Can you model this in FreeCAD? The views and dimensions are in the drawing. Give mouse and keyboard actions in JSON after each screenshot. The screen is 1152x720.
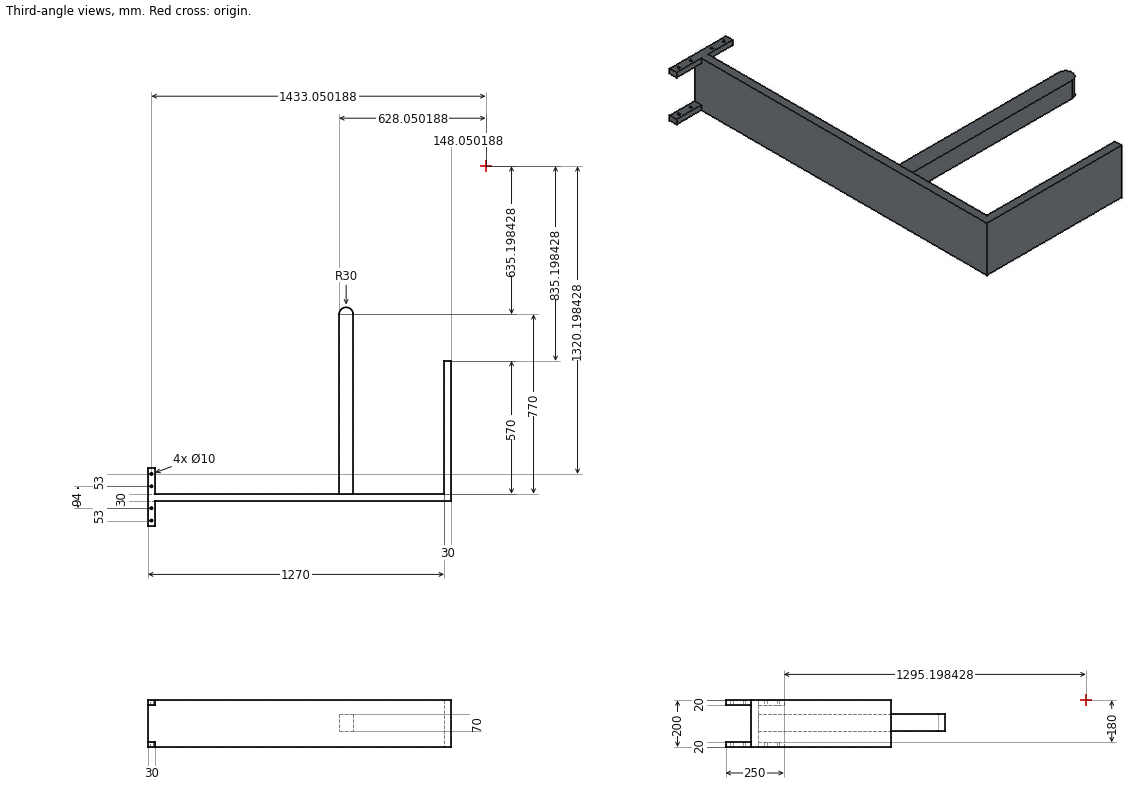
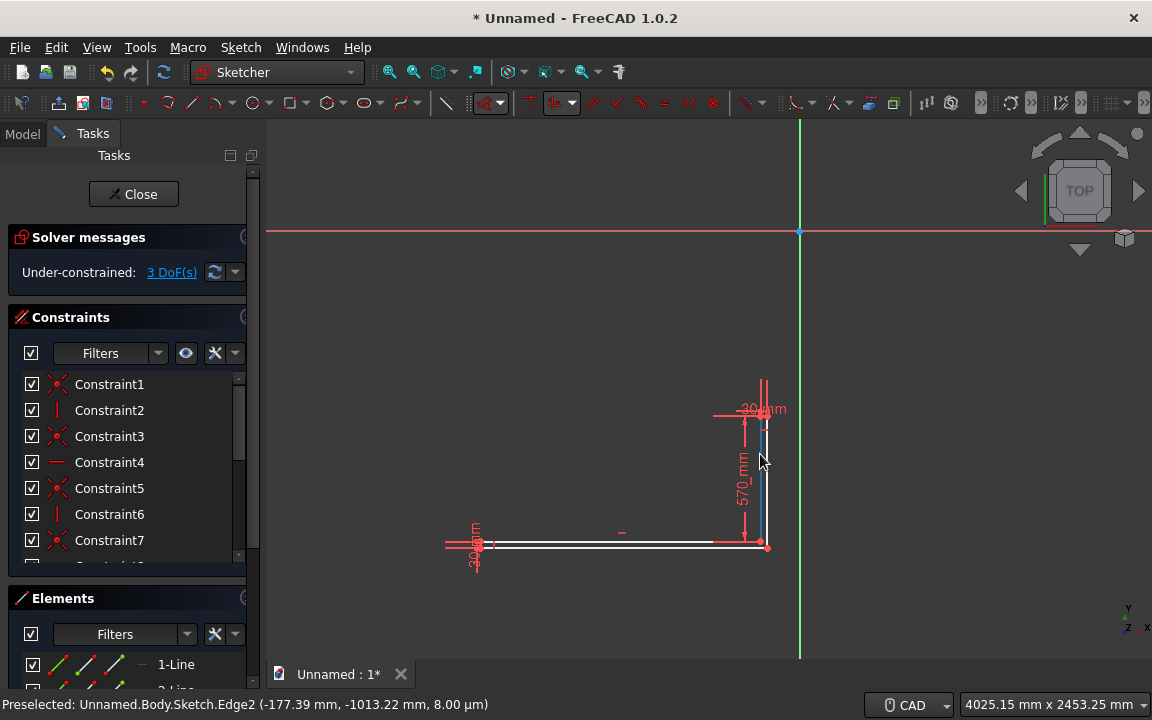
{"action": "scroll", "coordinate": [677, 542], "scroll_direction": "up", "scroll_amount": 4}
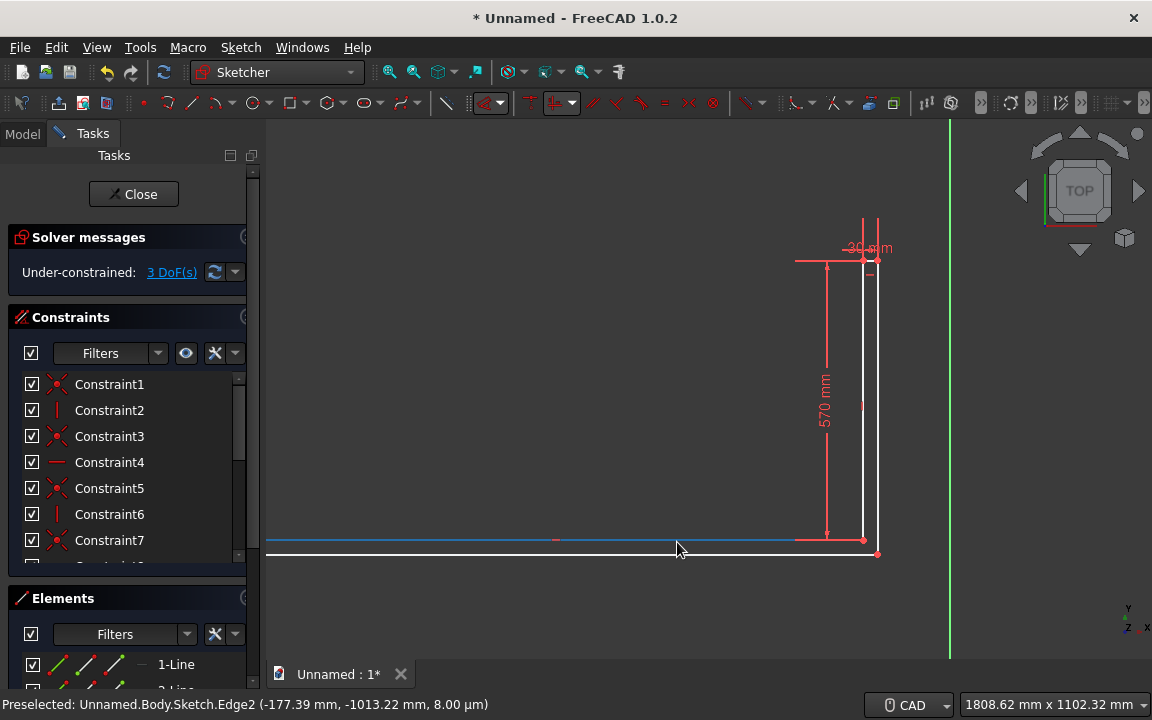
{"action": "left_click", "coordinate": [676, 540]}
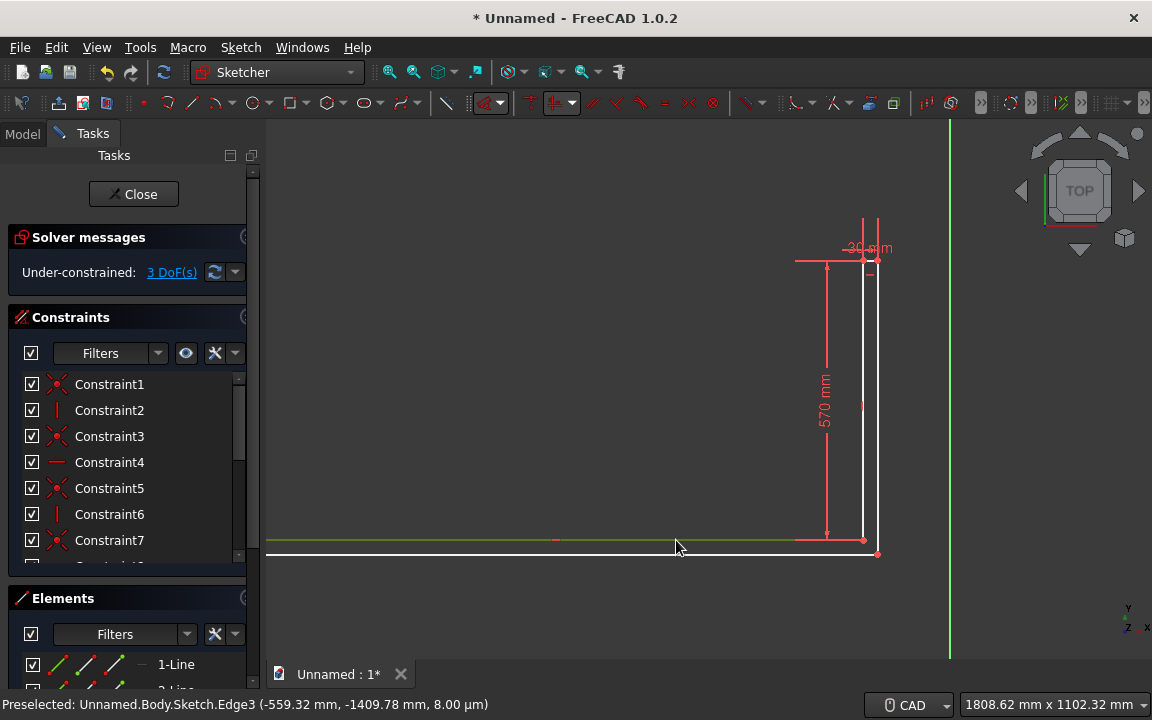
{"action": "left_click", "coordinate": [502, 104]}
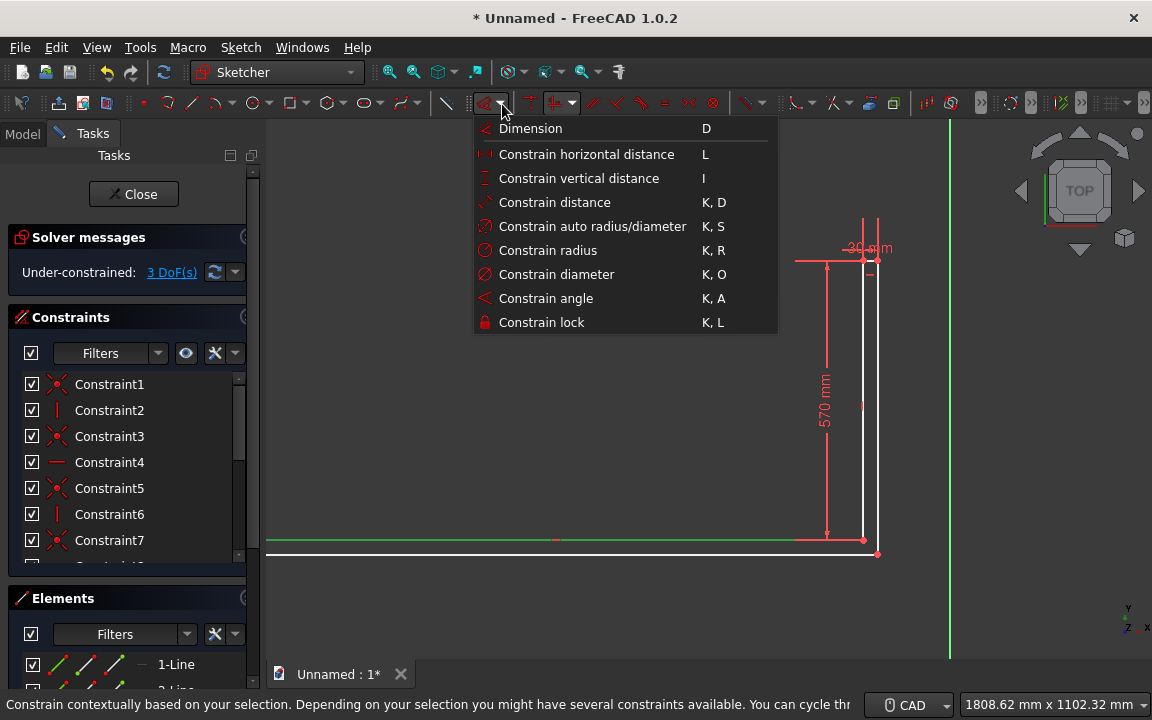
{"action": "left_click", "coordinate": [626, 154]}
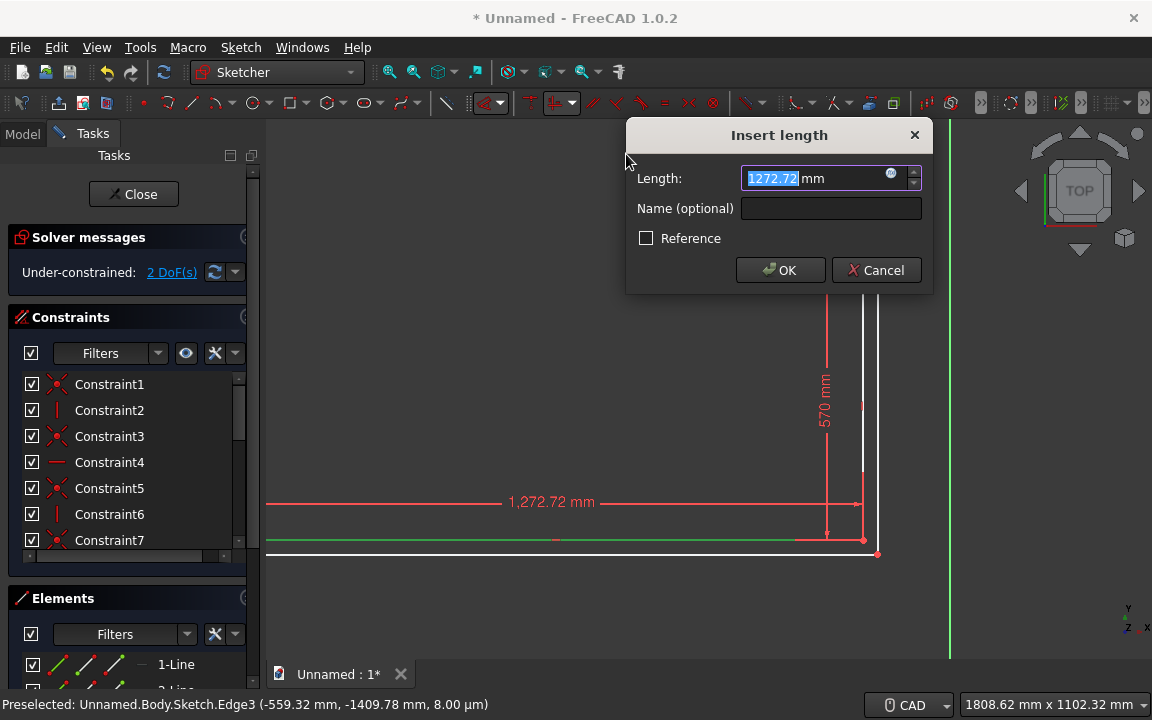
{"action": "type", "text": "1270"}
{"action": "key", "text": "Return"}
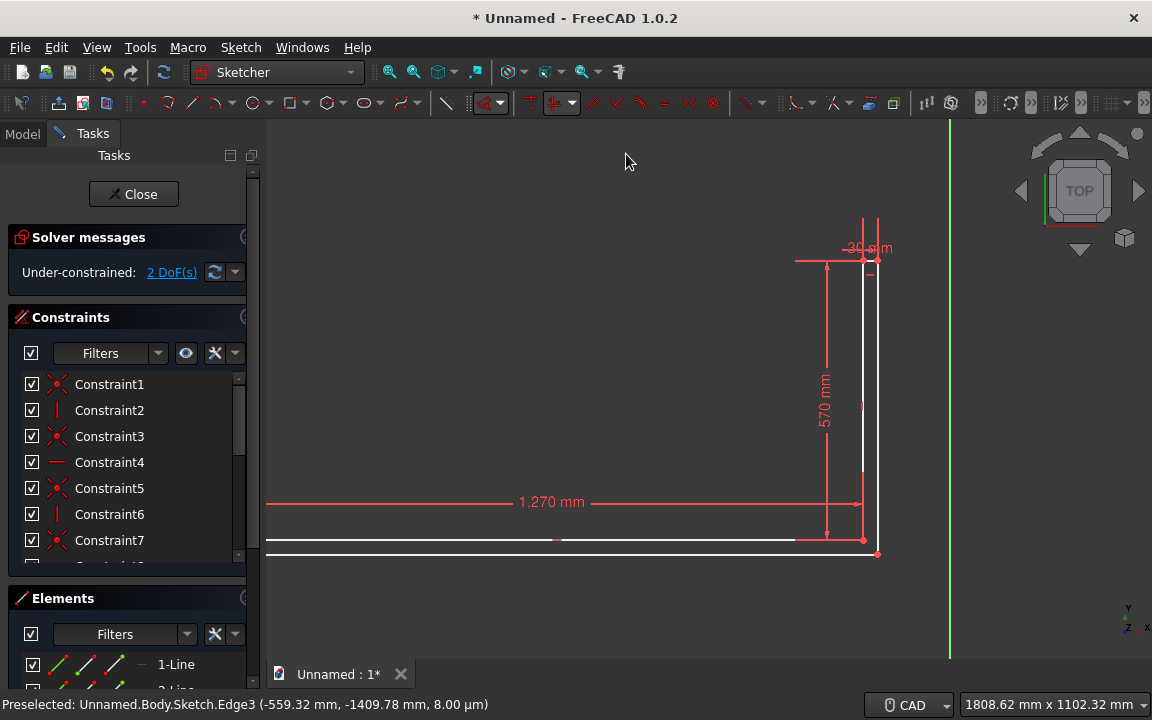
{"action": "left_click", "coordinate": [878, 261]}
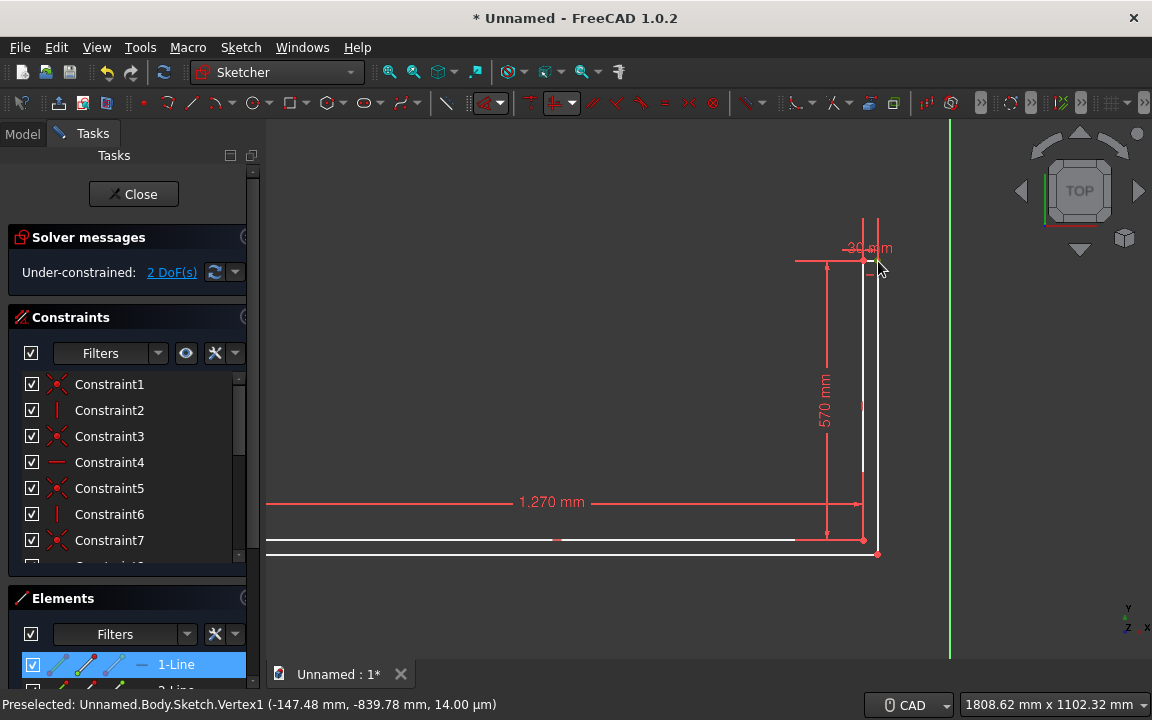
{"action": "key", "text": "l"}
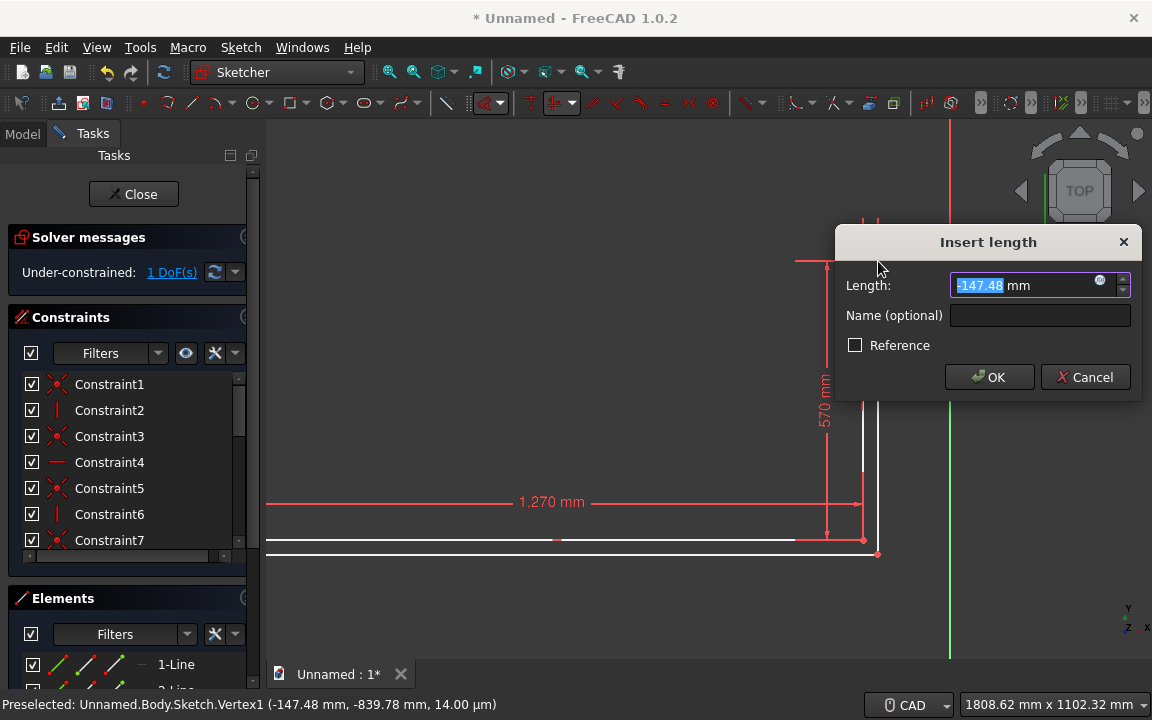
{"action": "type", "text": "-148.050188"}
{"action": "key", "text": "Return"}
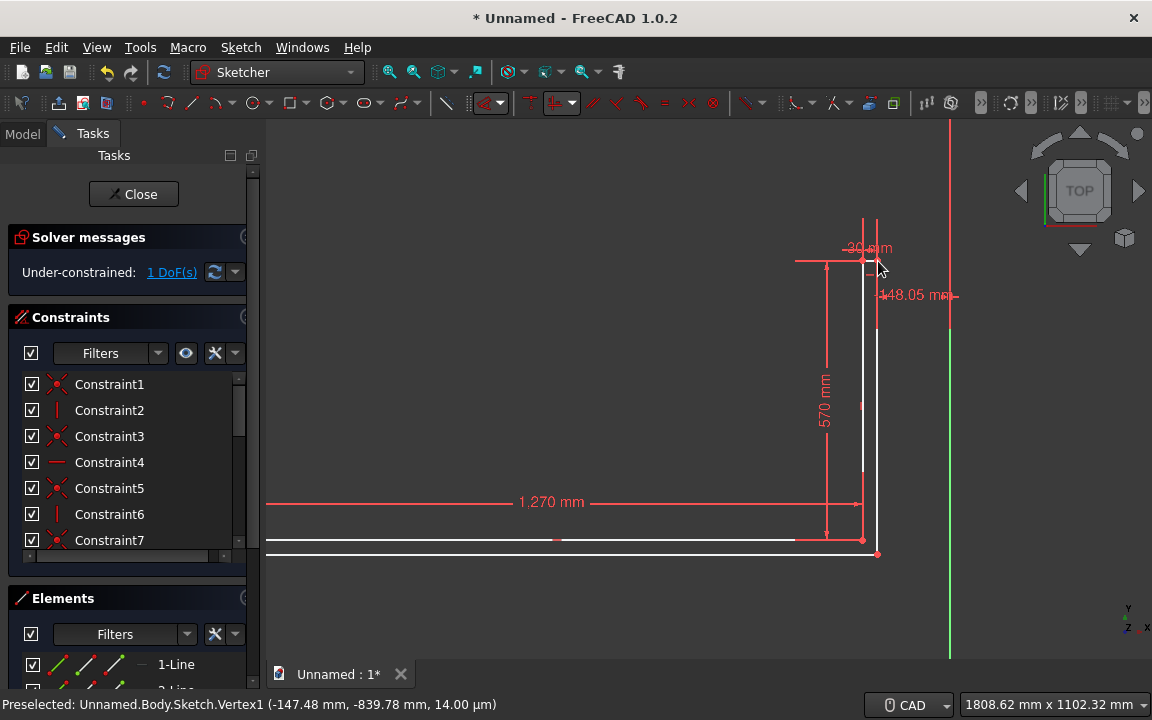
{"action": "left_click", "coordinate": [877, 261]}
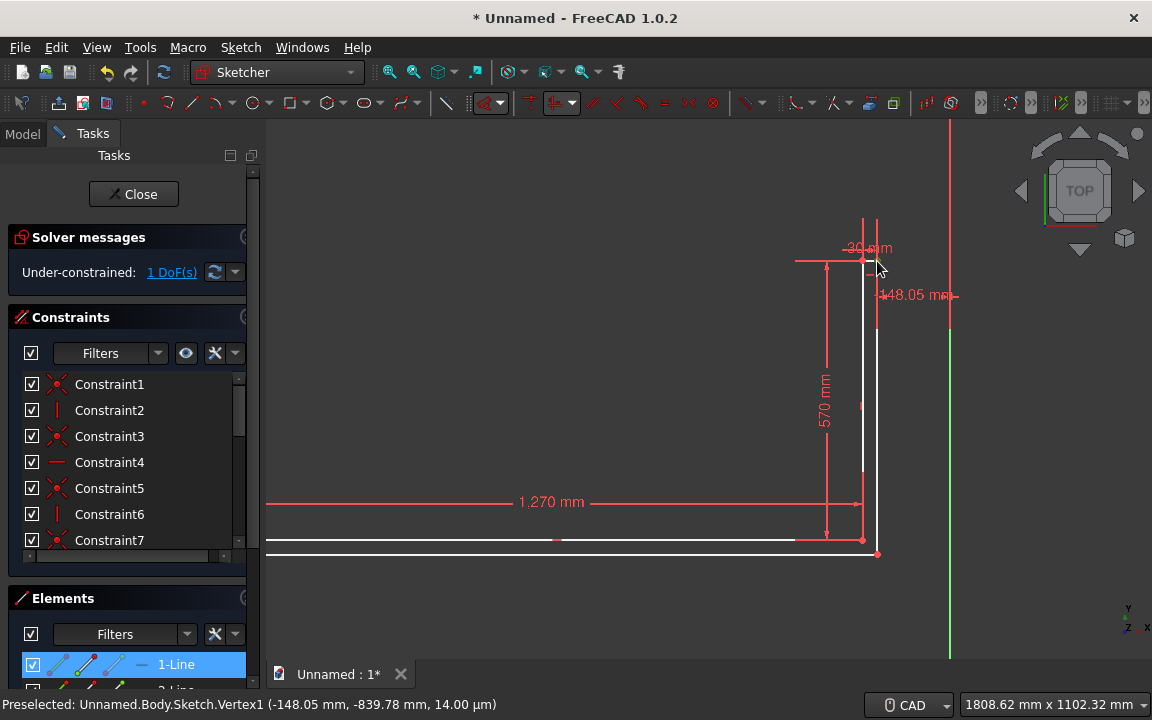
{"action": "key", "text": "i"}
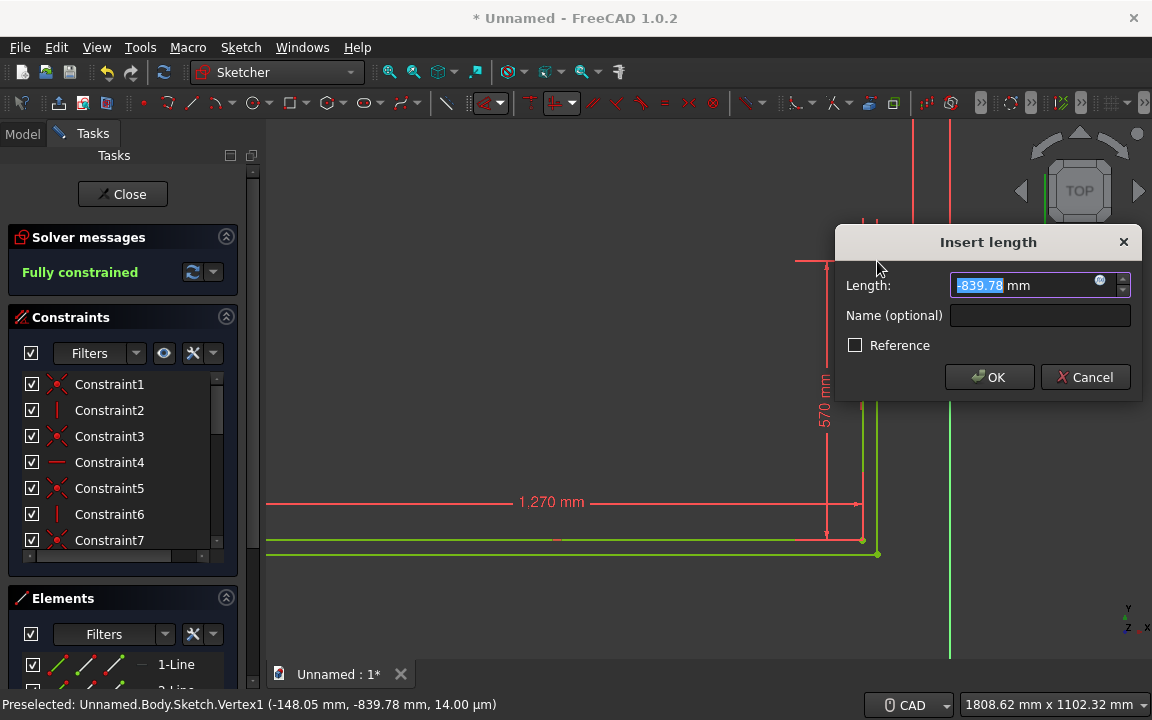
{"action": "type", "text": "-835.198428"}
{"action": "key", "text": "Return"}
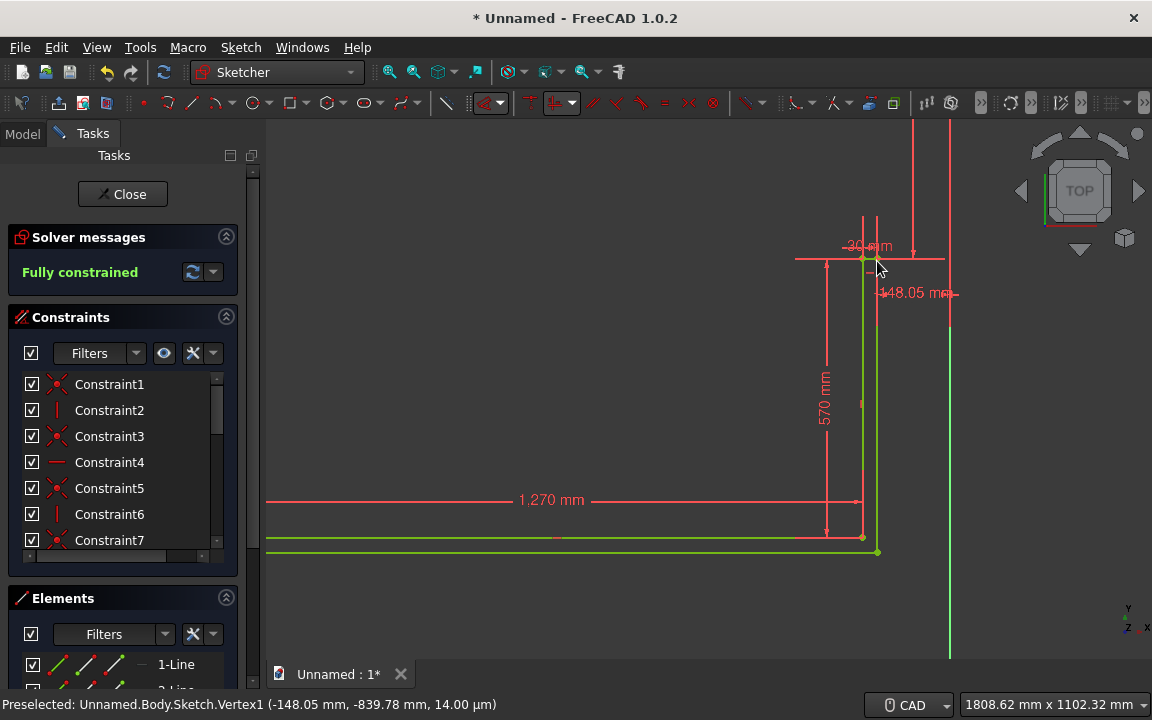
{"action": "left_click", "coordinate": [123, 194]}